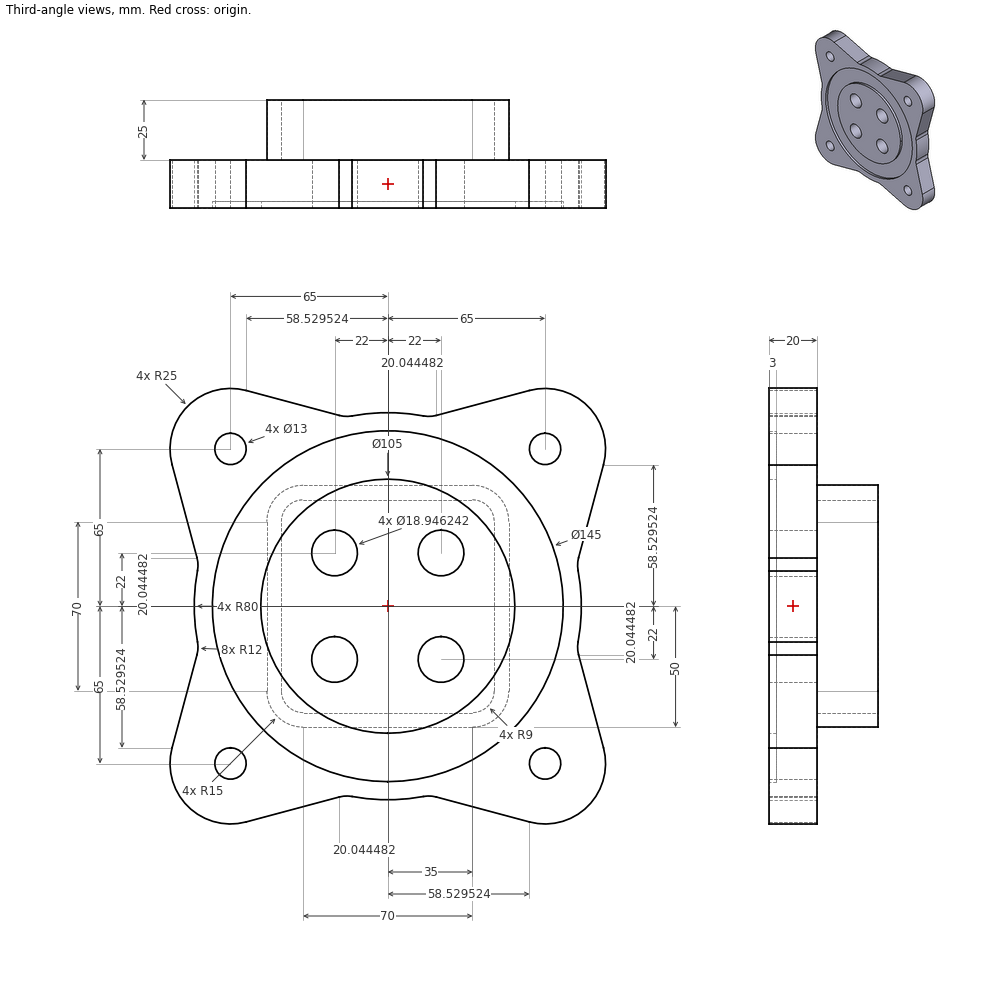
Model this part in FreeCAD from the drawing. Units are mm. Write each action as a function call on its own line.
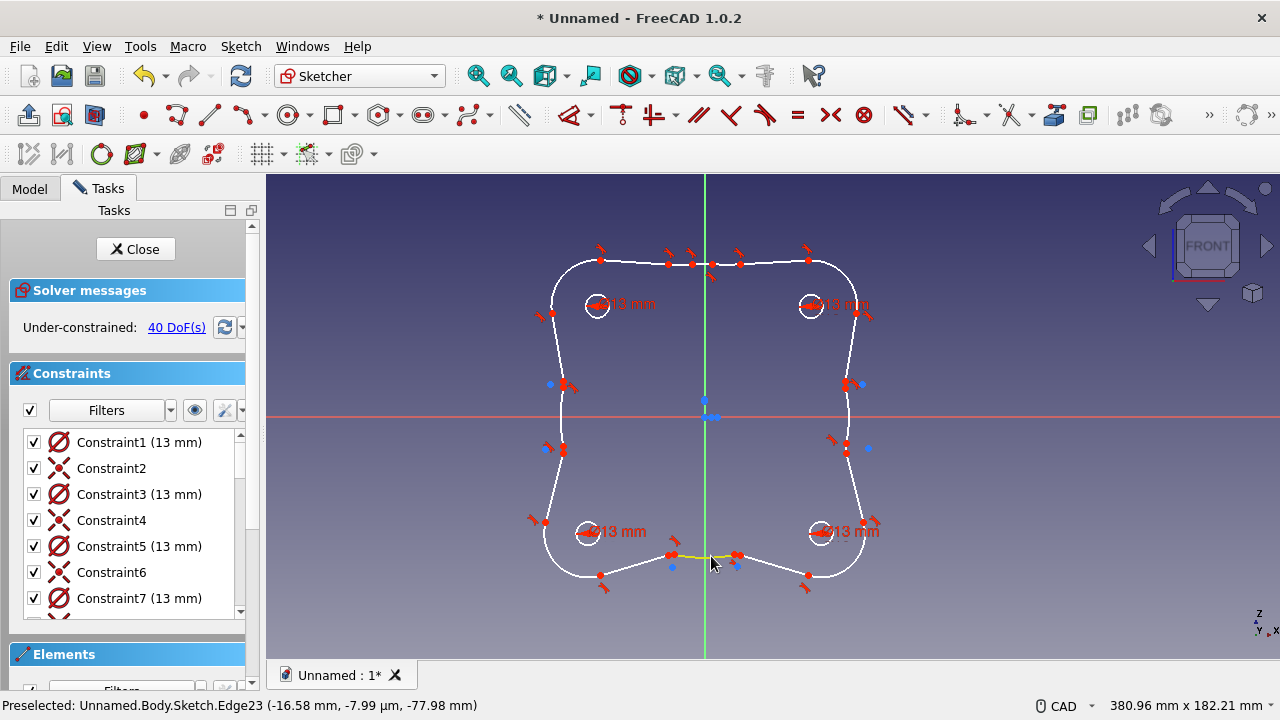
click(561, 405)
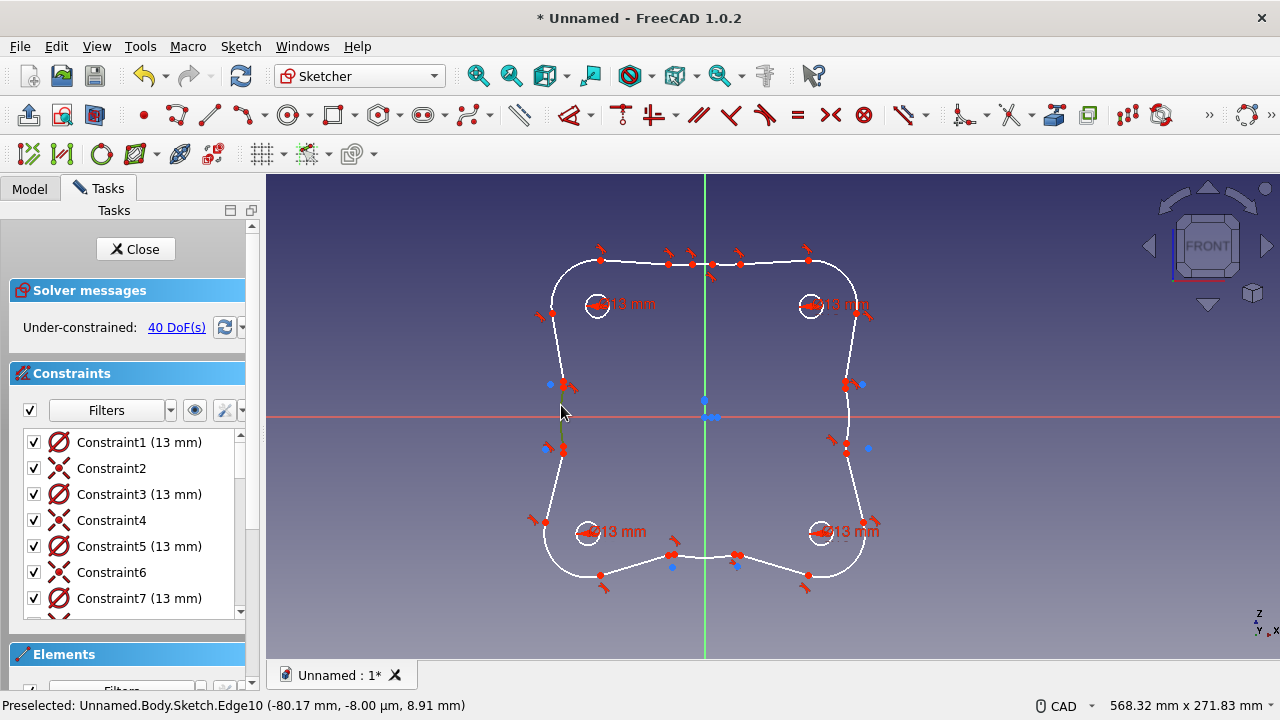
scroll(703, 264, up, 2)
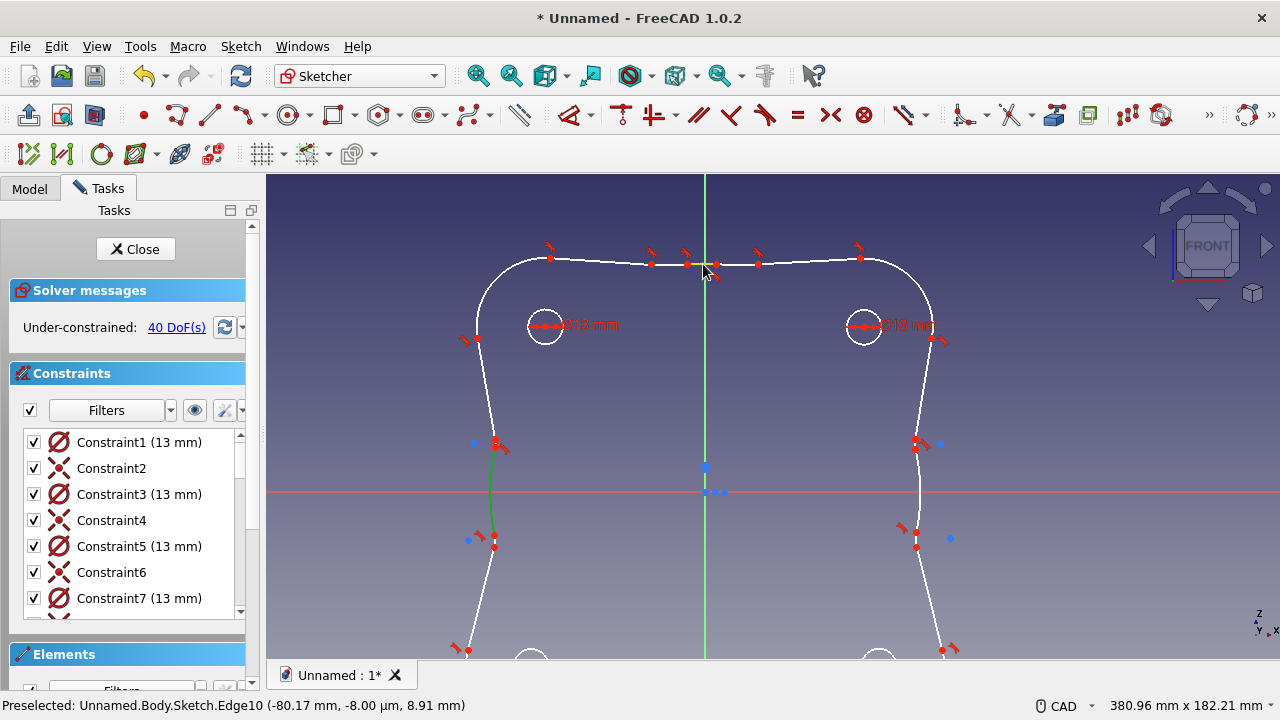
click(702, 264)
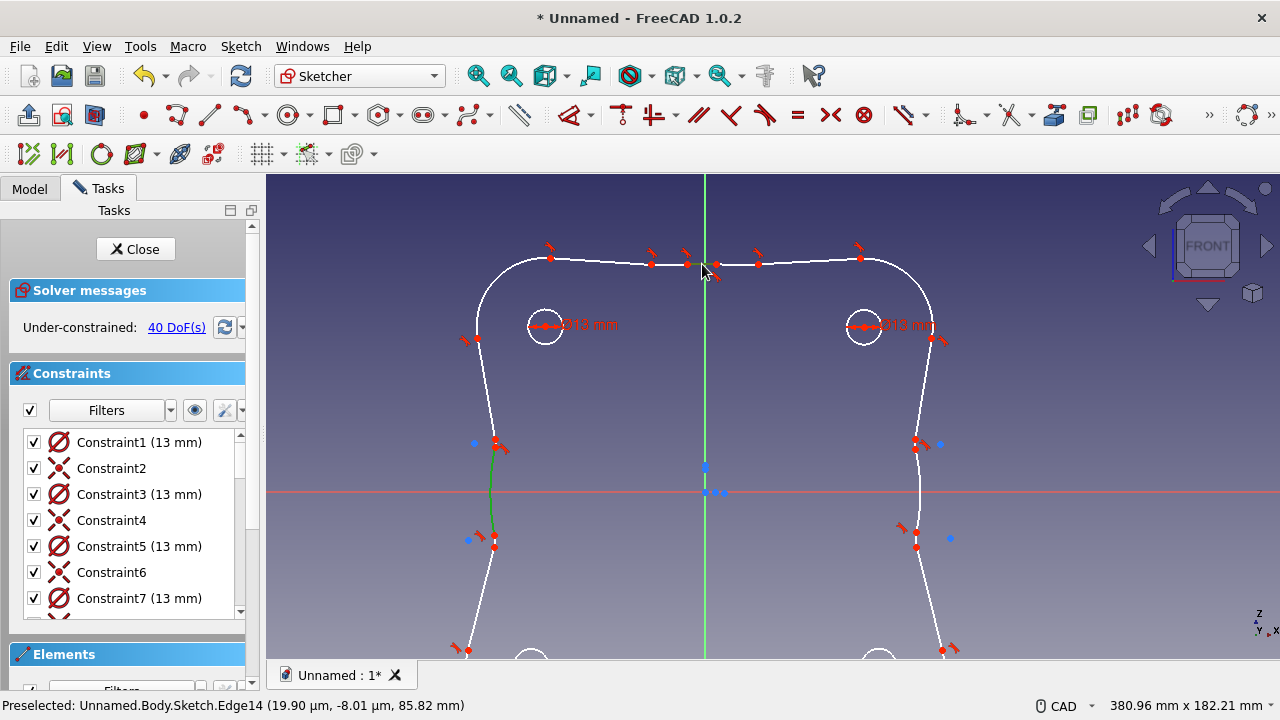
click(621, 116)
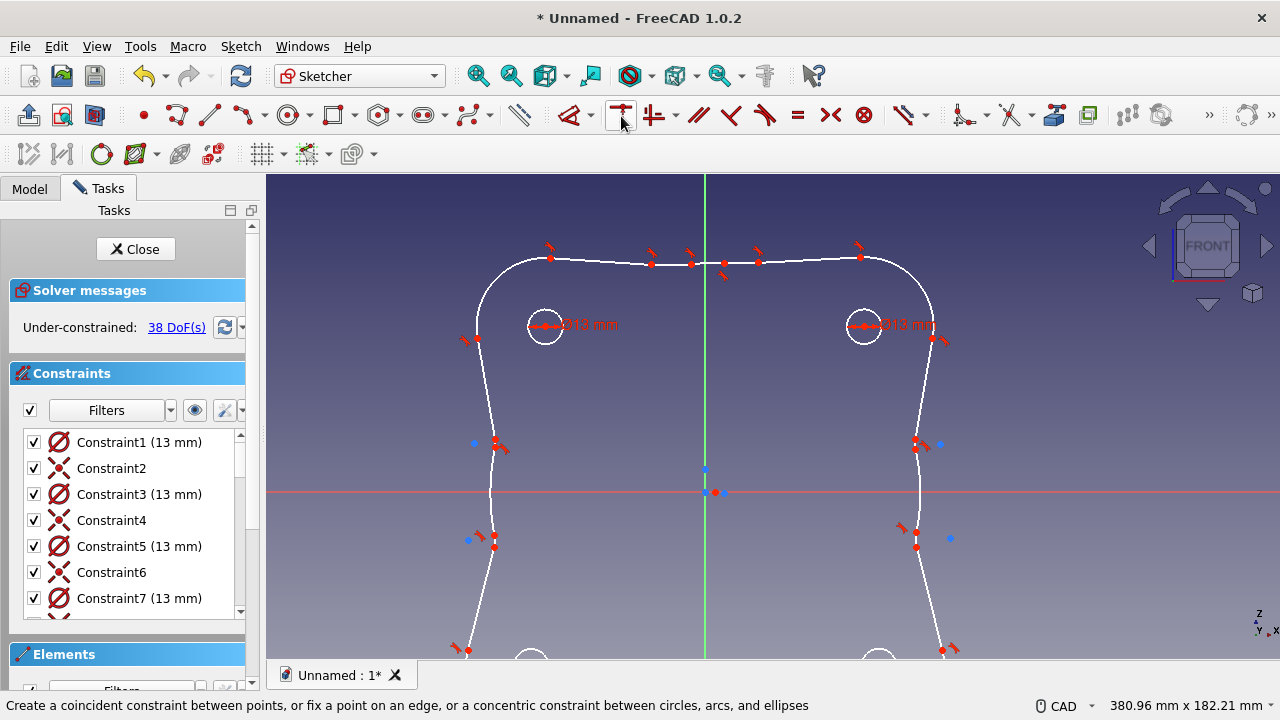
click(491, 474)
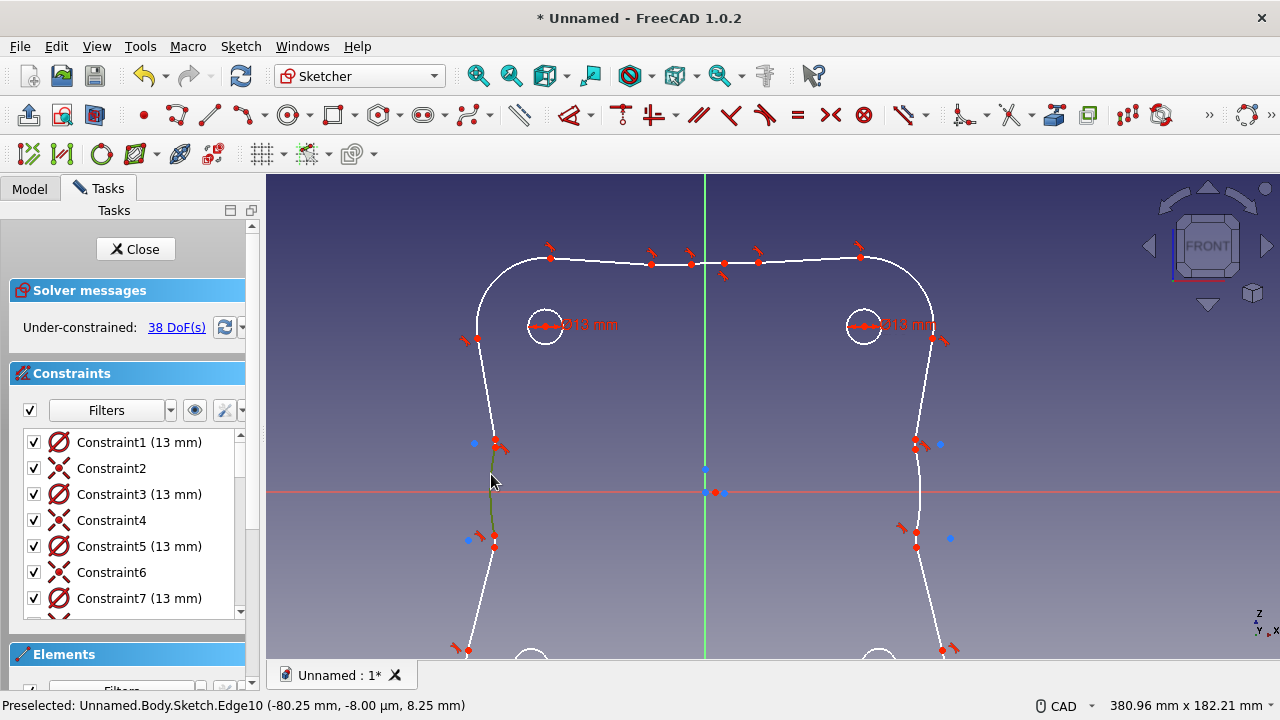
click(920, 508)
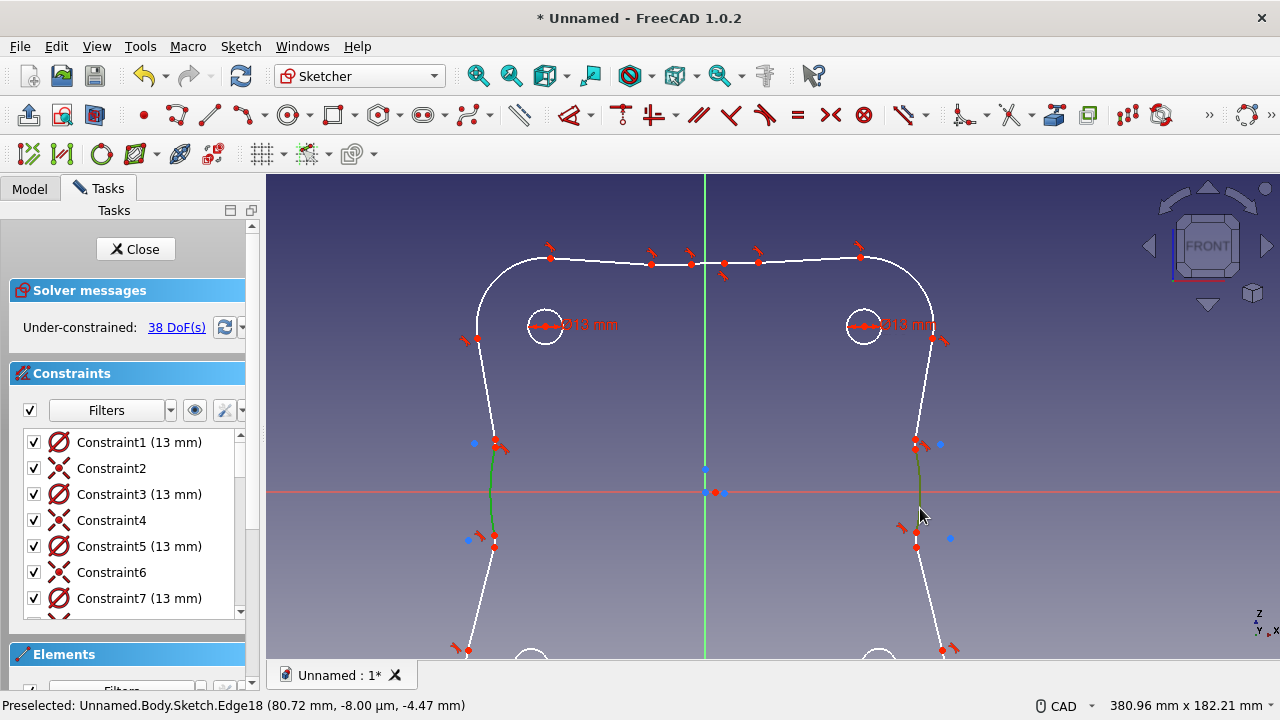
key(c)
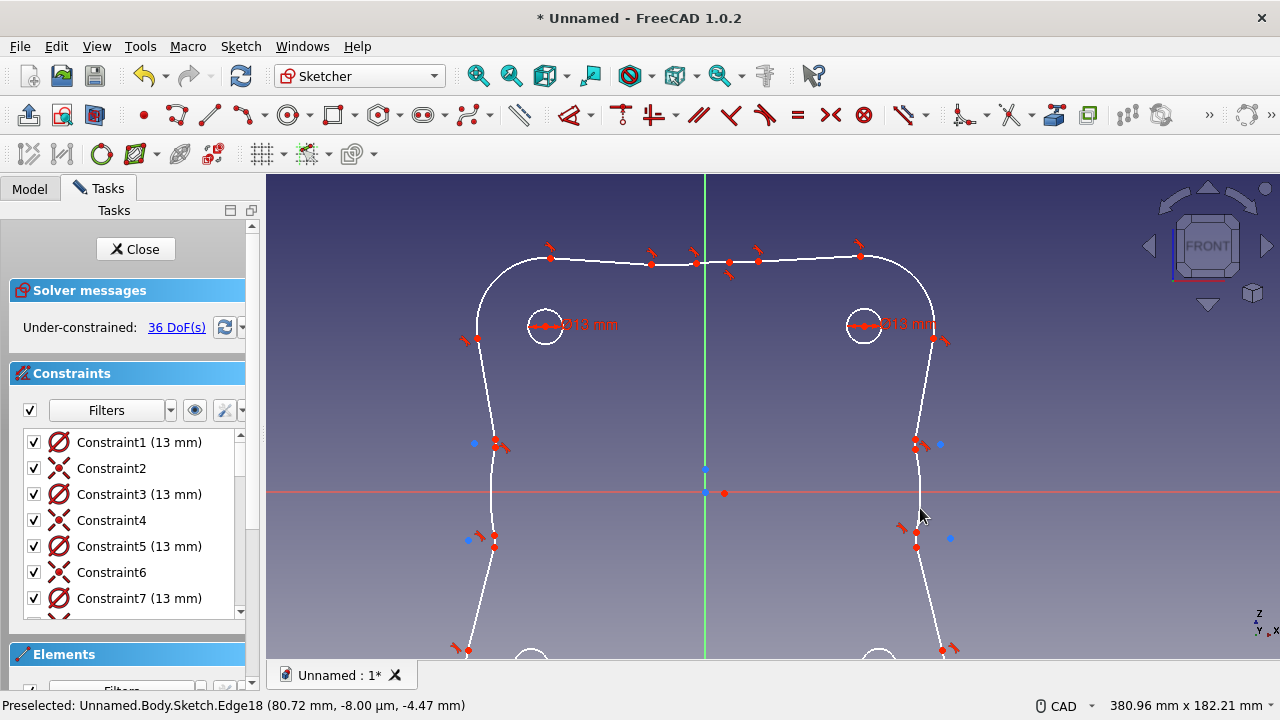
click(491, 474)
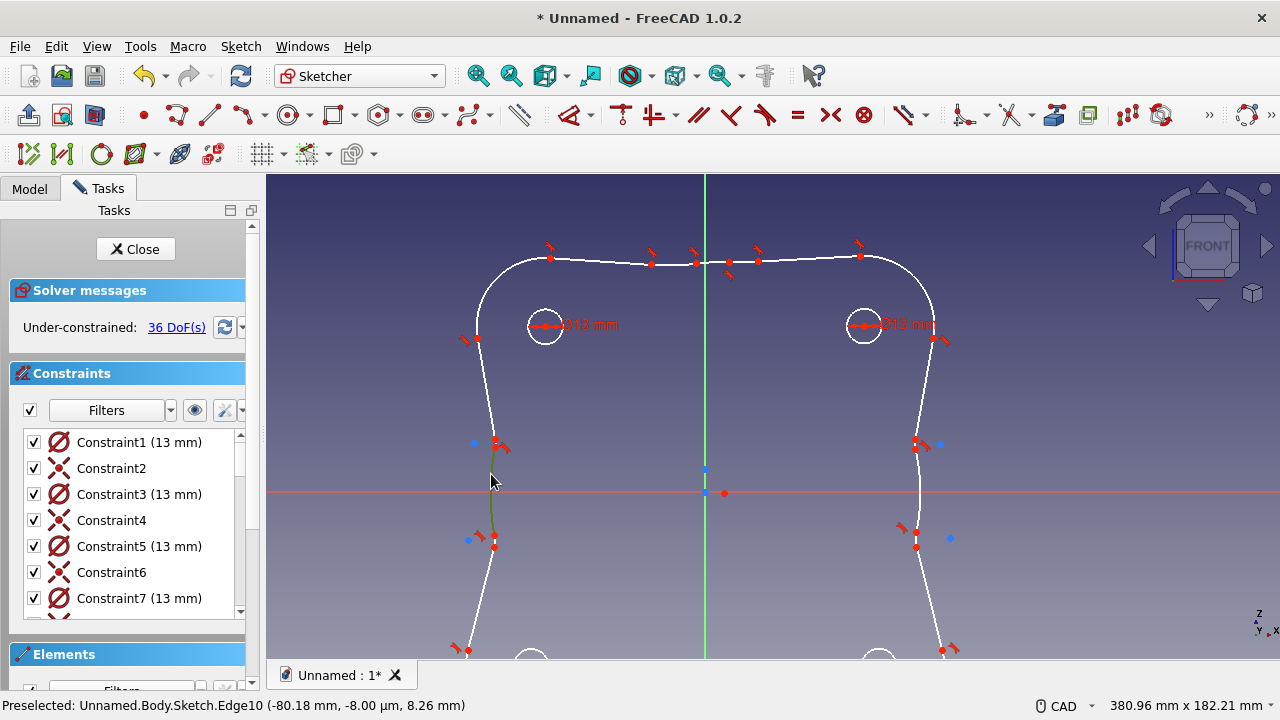
scroll(703, 262, down, 2)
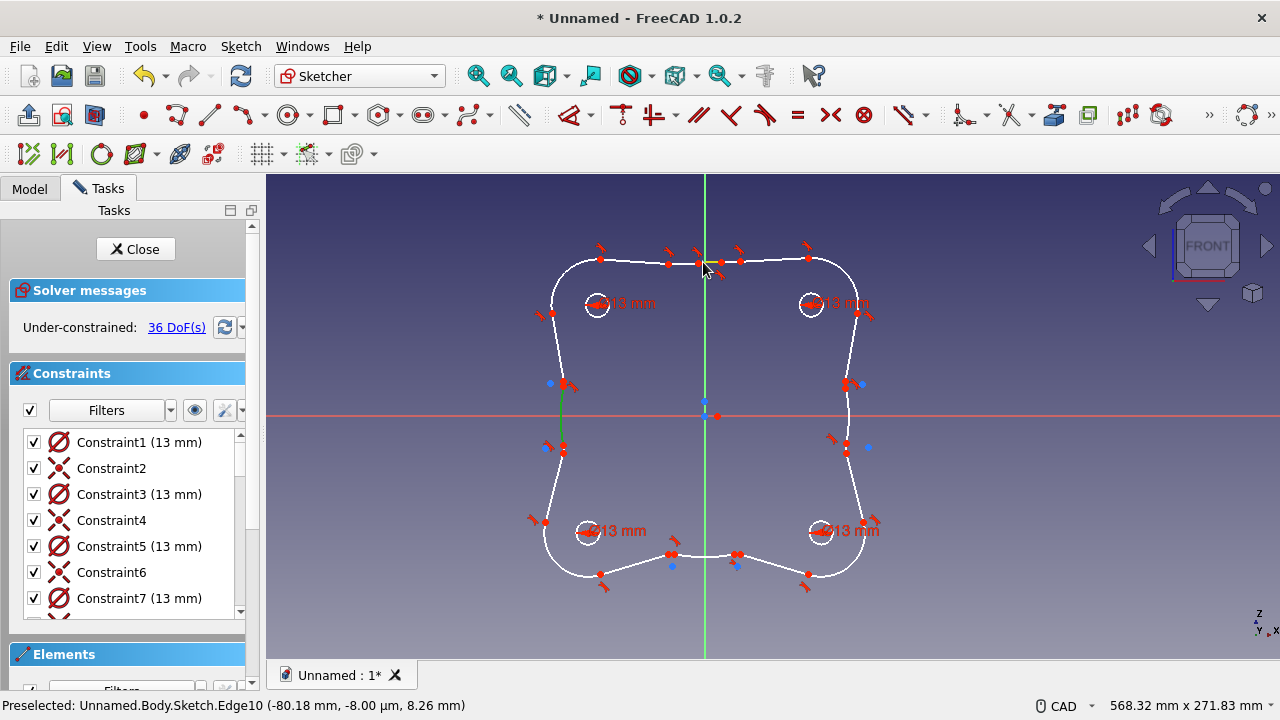
click(693, 557)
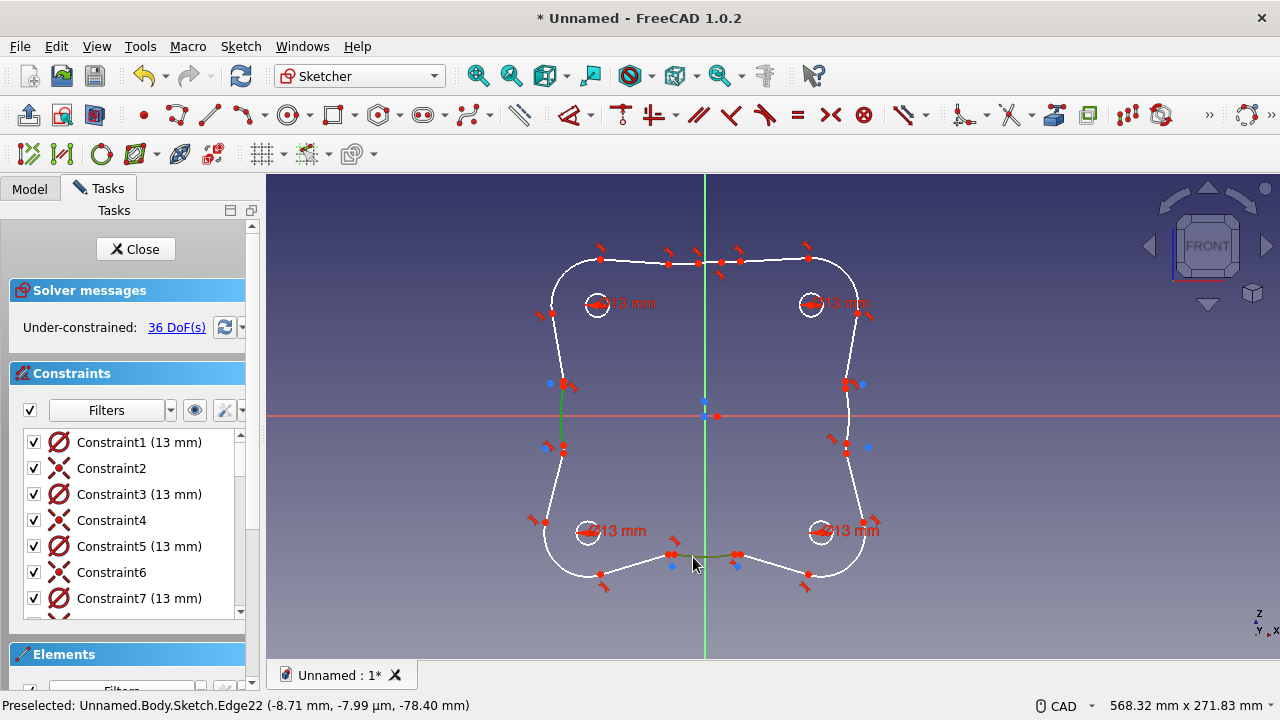
click(621, 116)